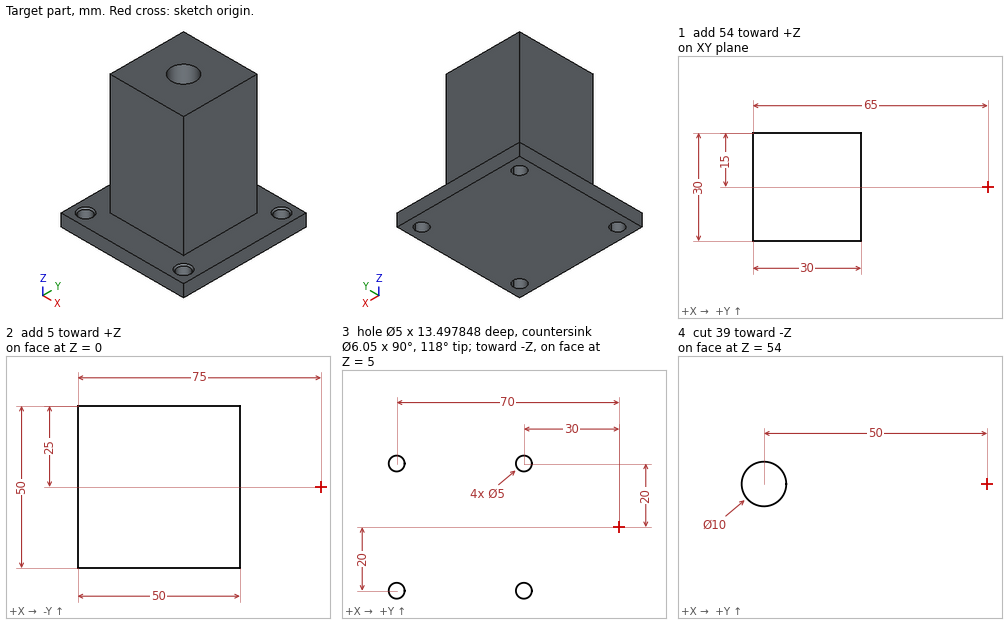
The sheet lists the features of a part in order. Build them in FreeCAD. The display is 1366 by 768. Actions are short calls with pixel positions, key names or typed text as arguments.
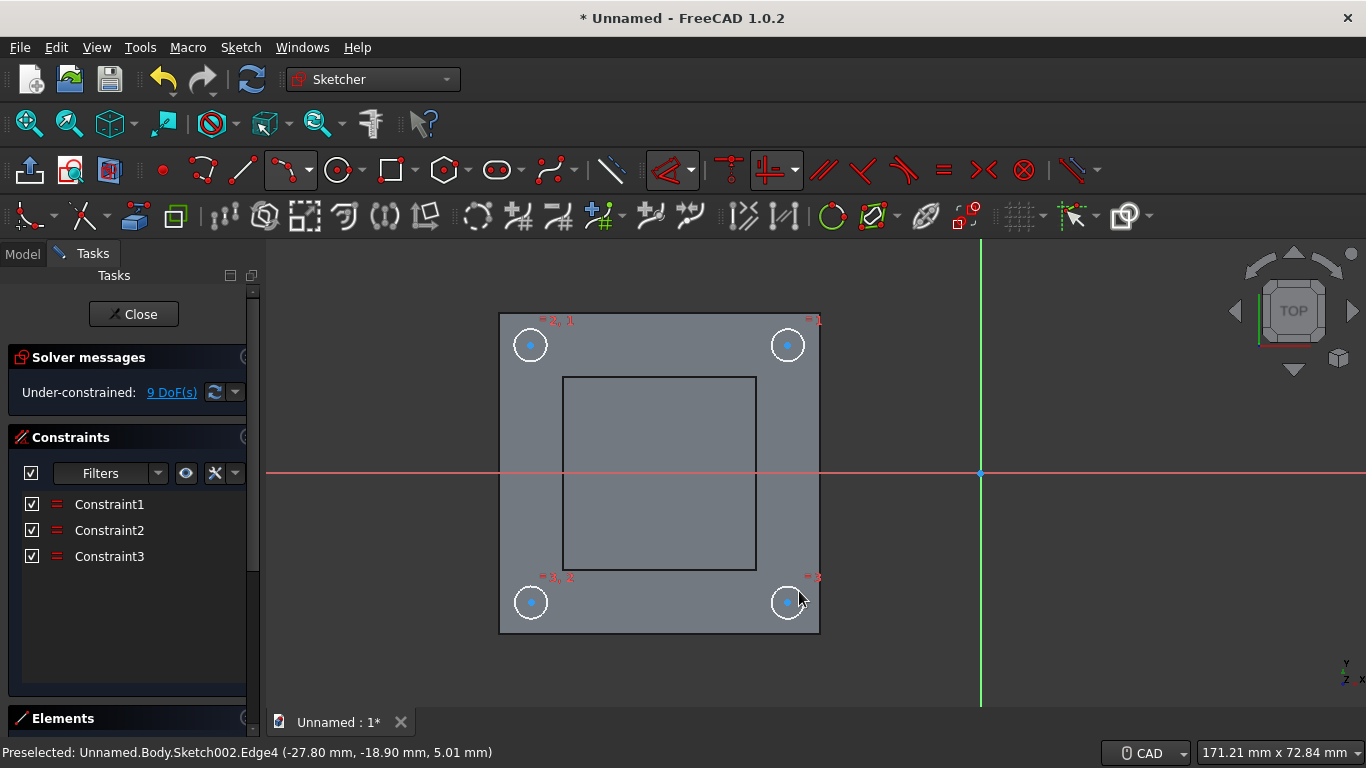
click(788, 345)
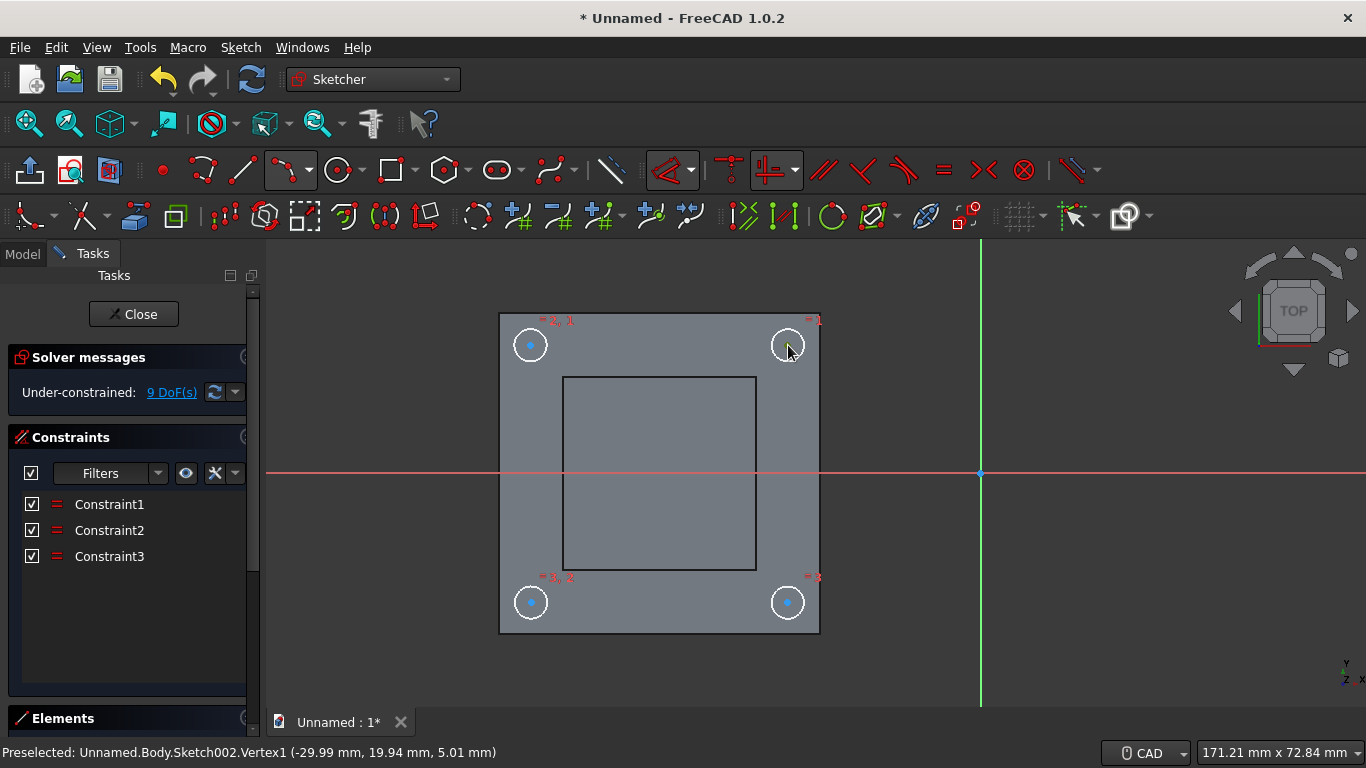
click(530, 345)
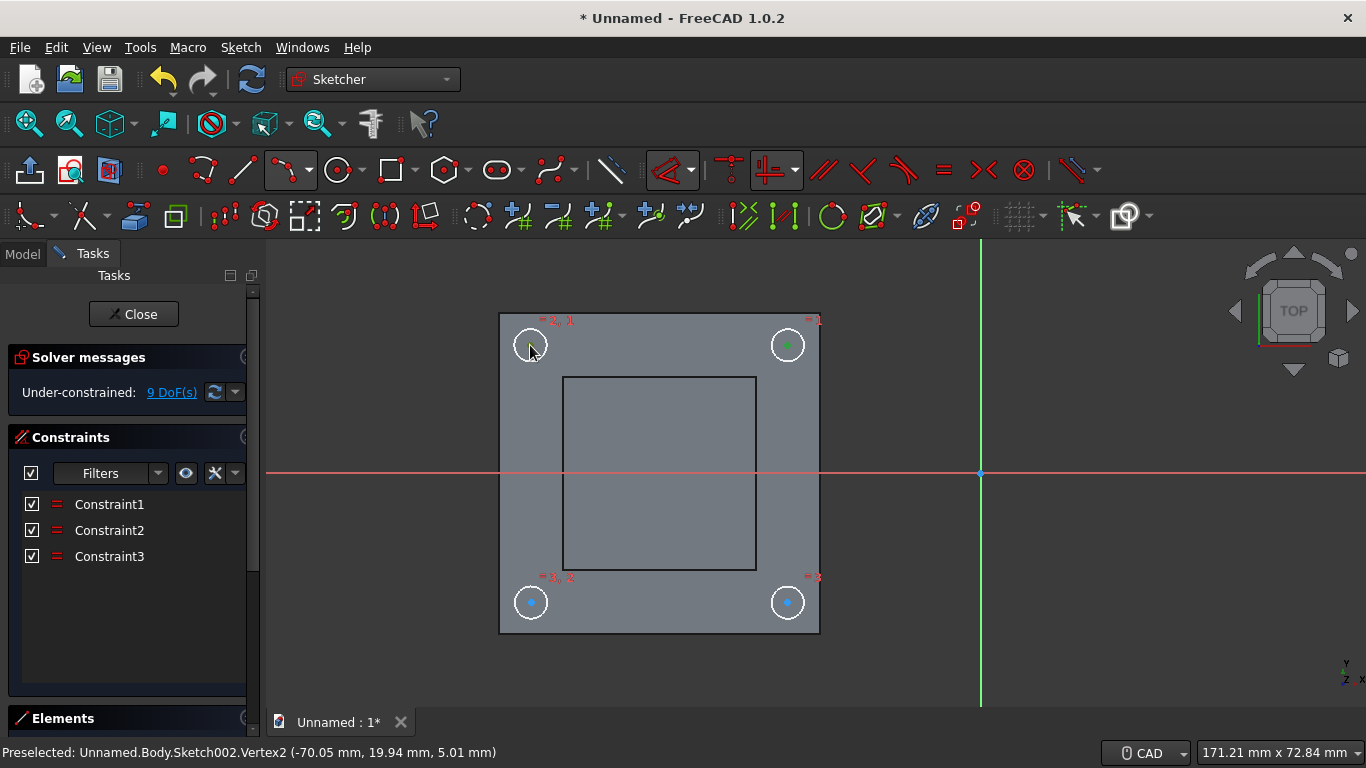
key(h)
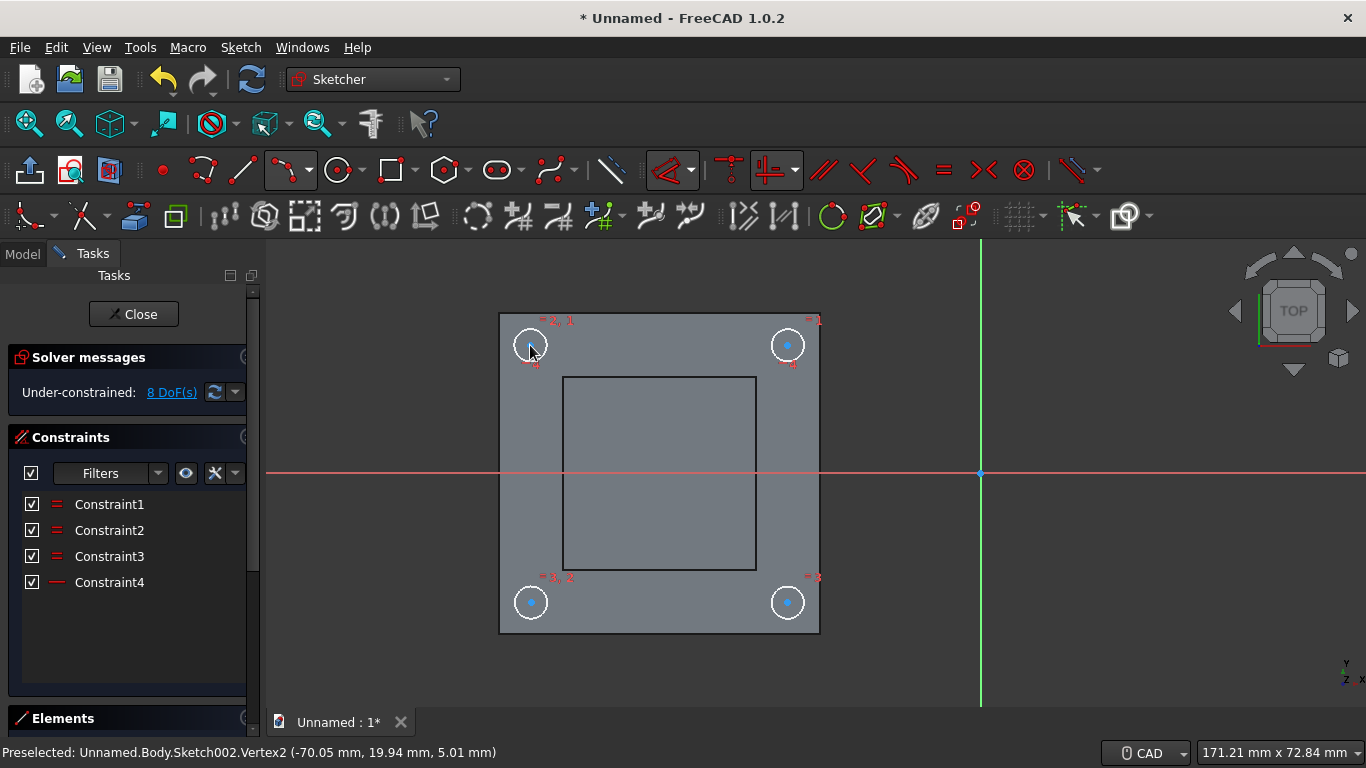
click(530, 345)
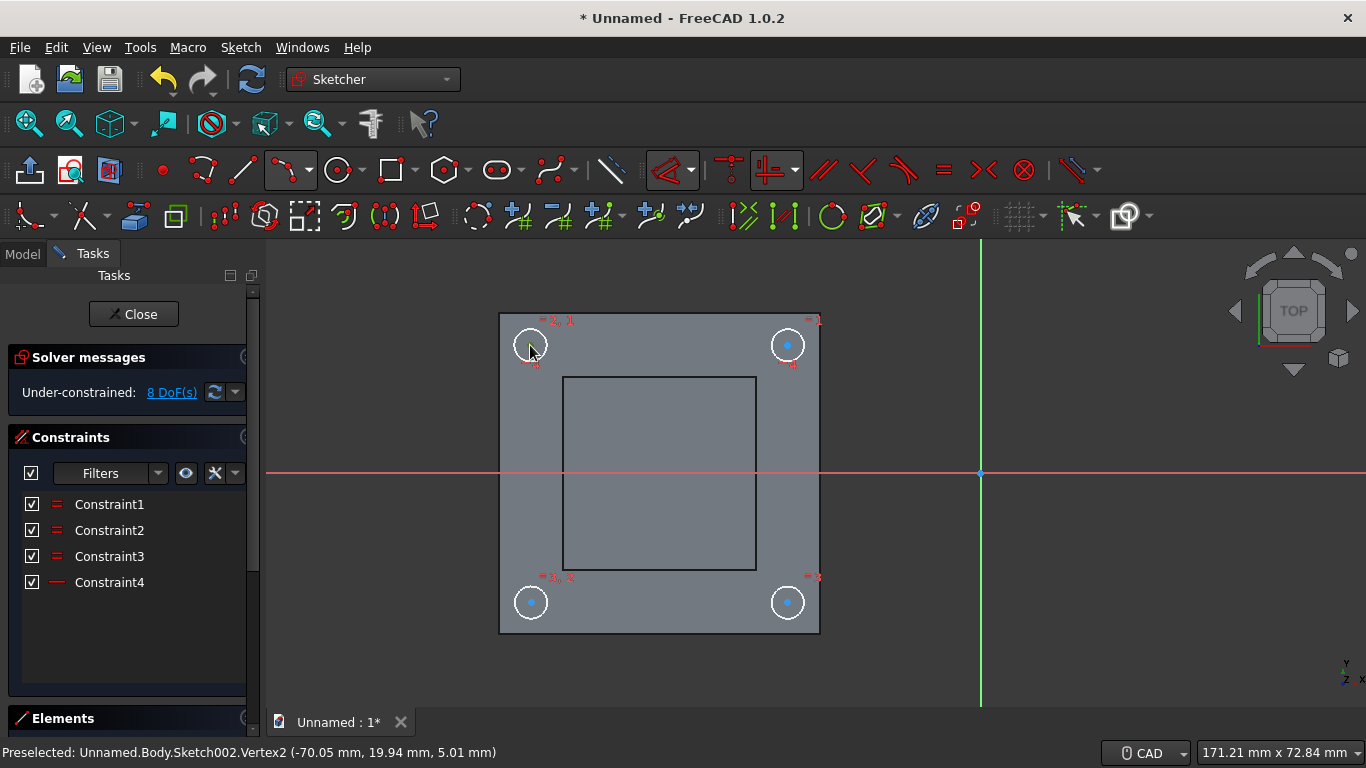
click(531, 603)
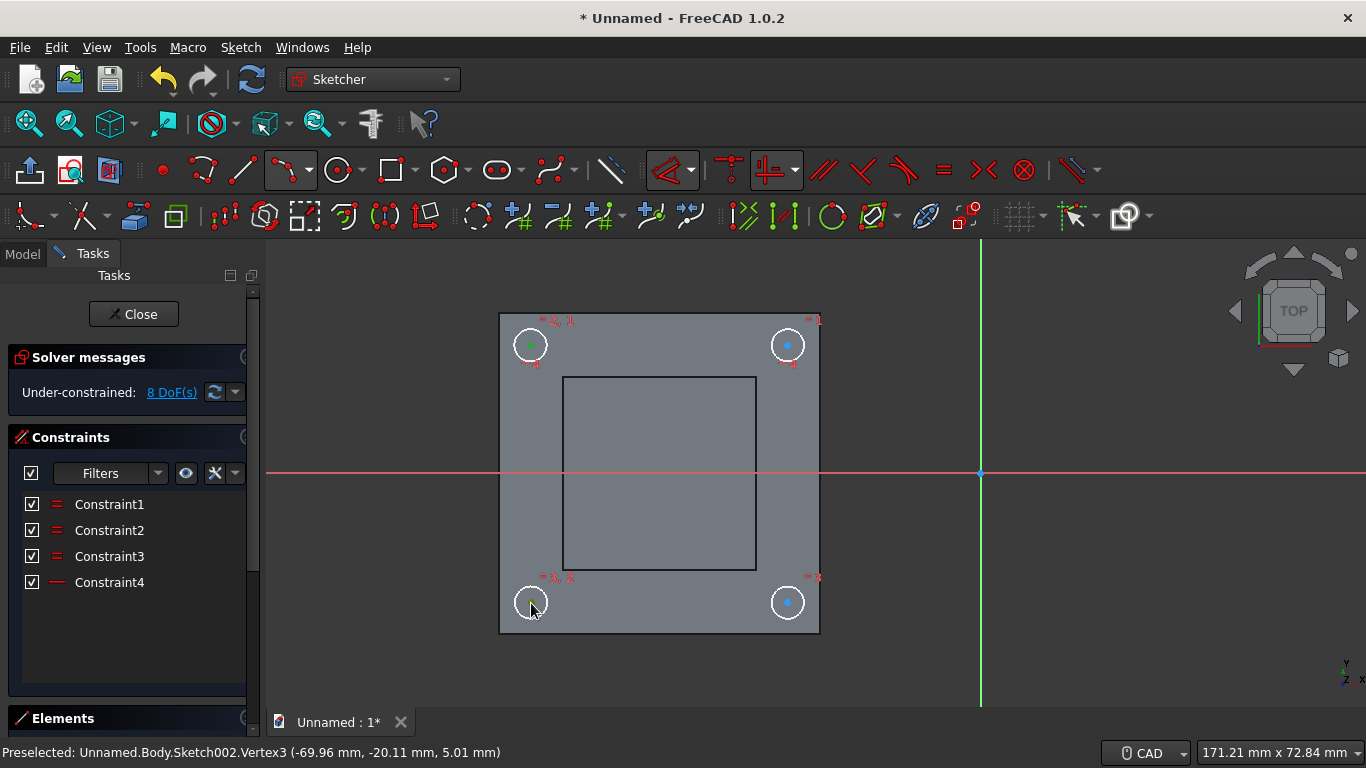
key(v)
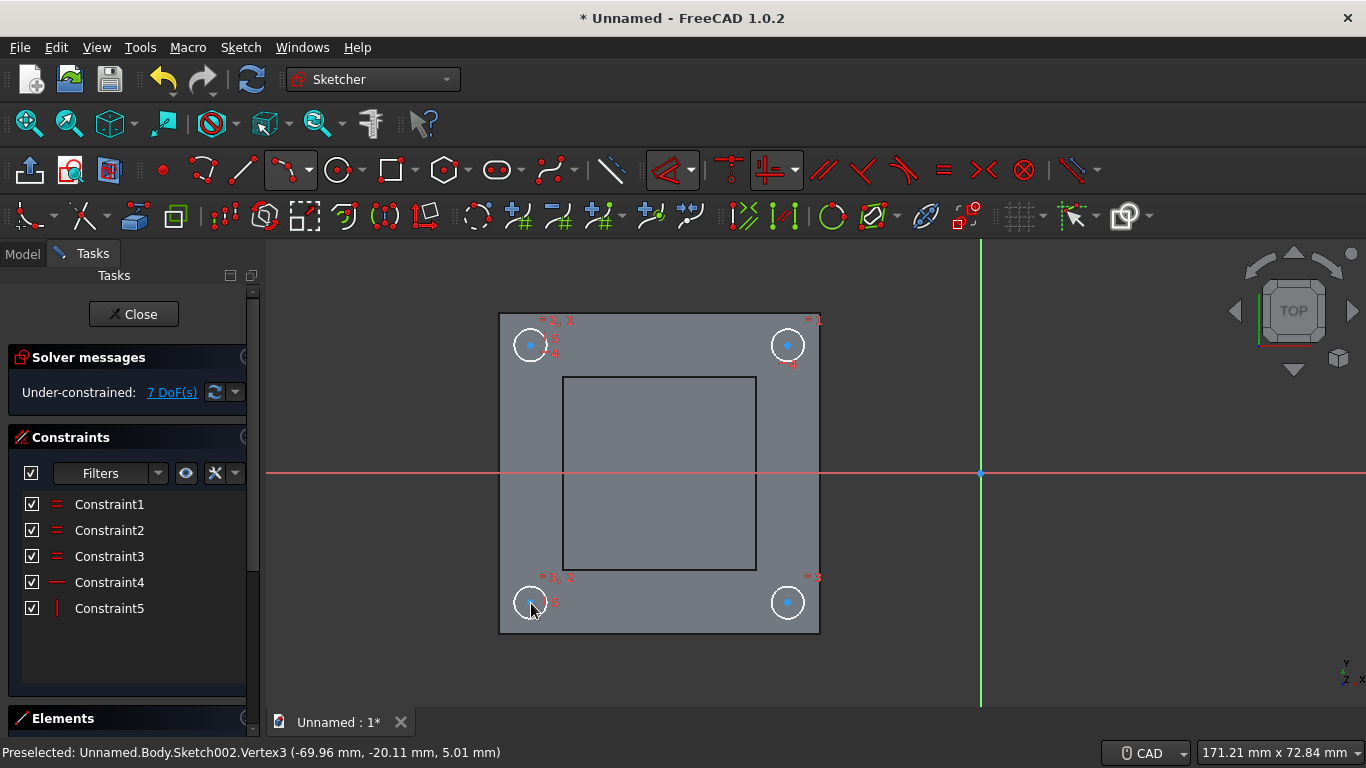
click(788, 345)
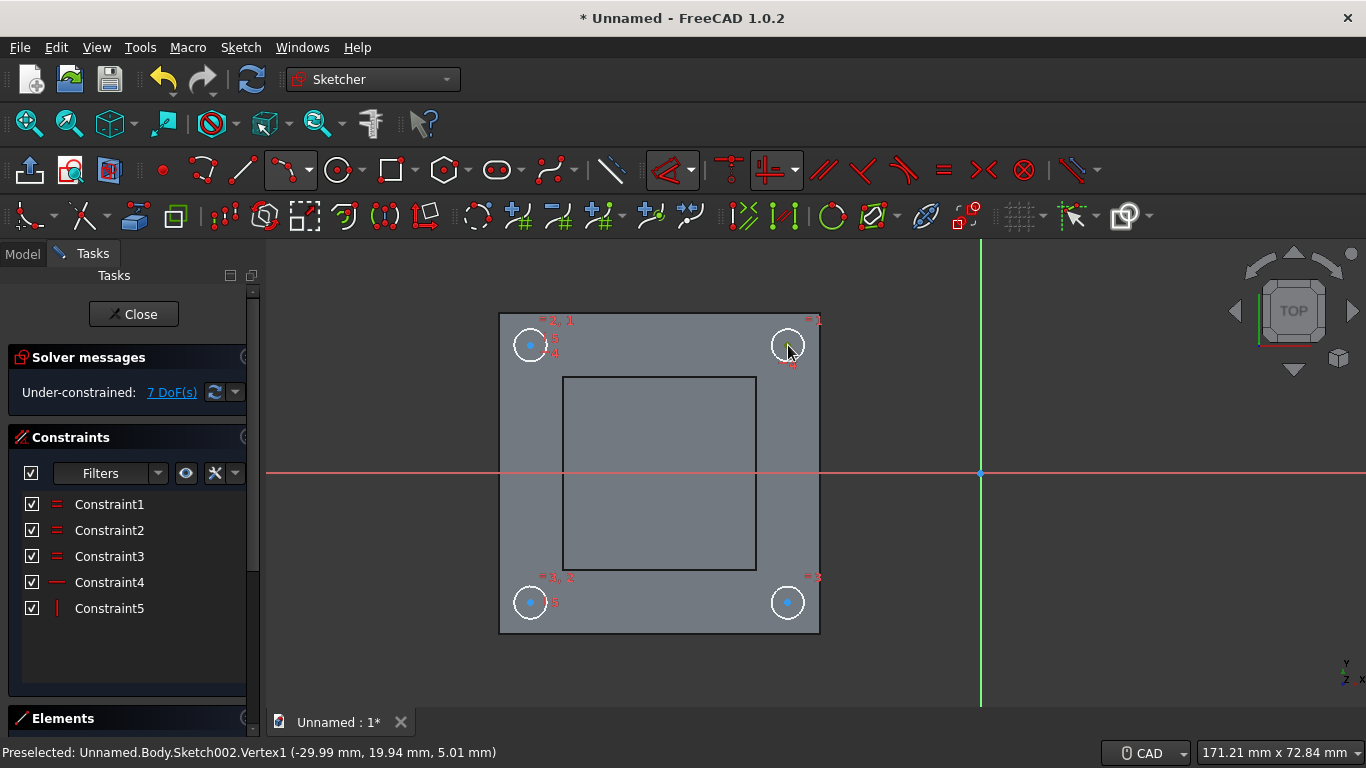
click(788, 603)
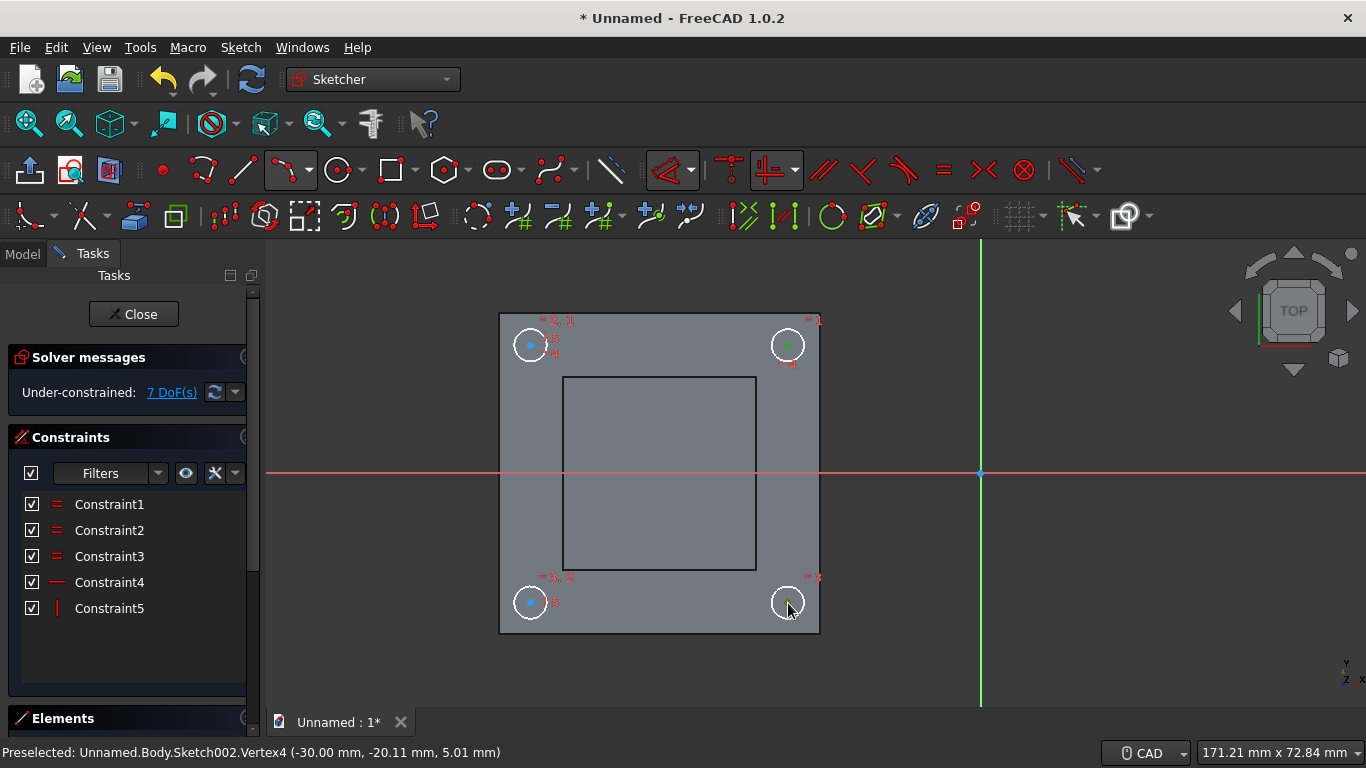
key(v)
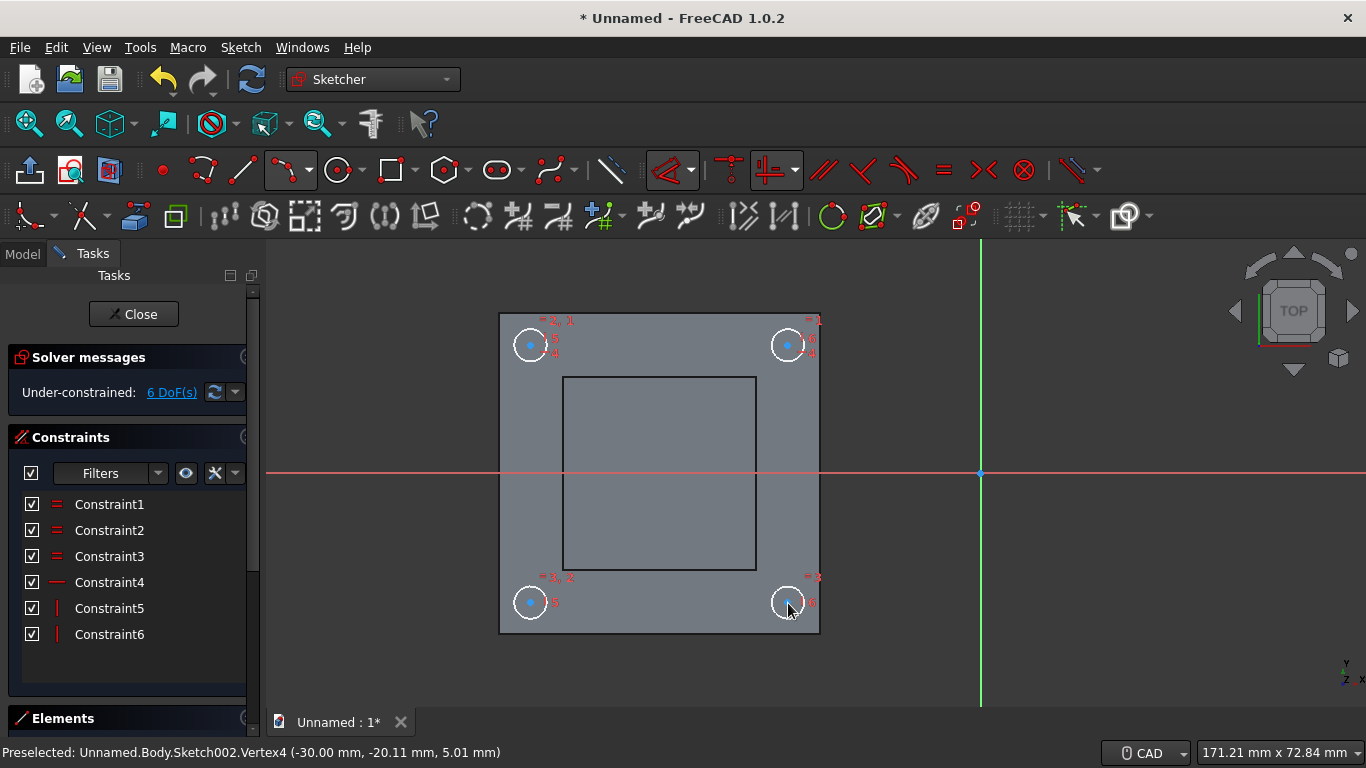
click(530, 603)